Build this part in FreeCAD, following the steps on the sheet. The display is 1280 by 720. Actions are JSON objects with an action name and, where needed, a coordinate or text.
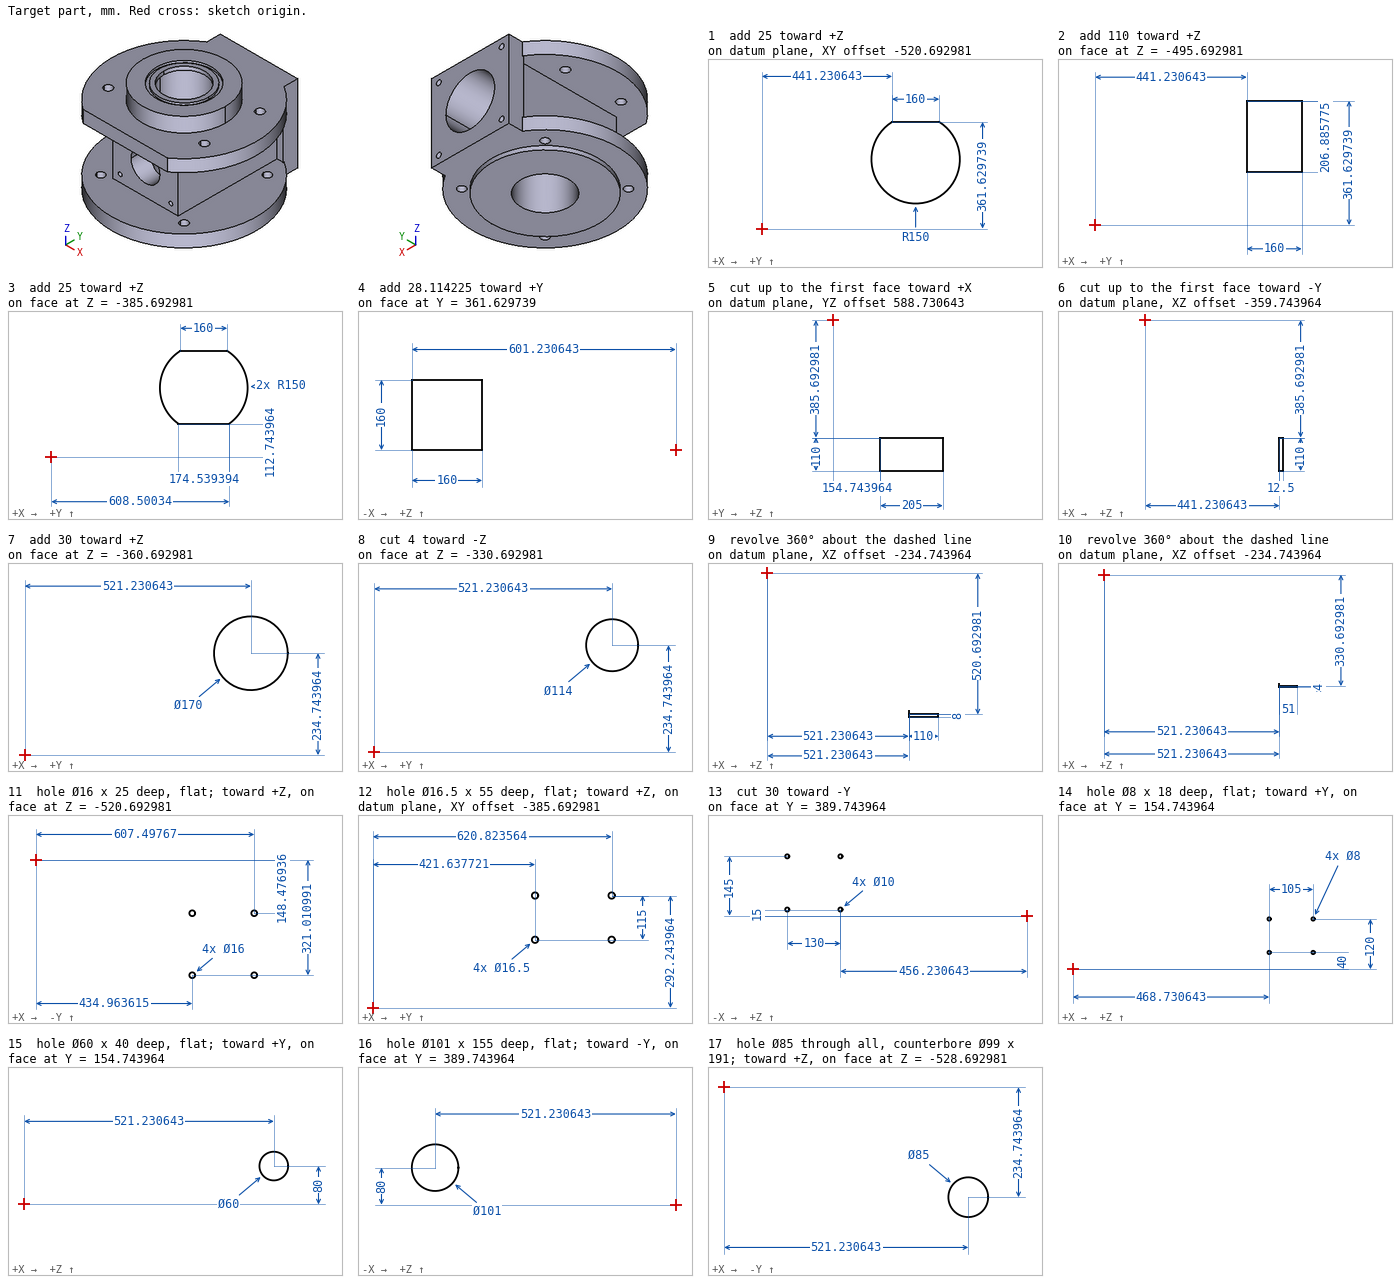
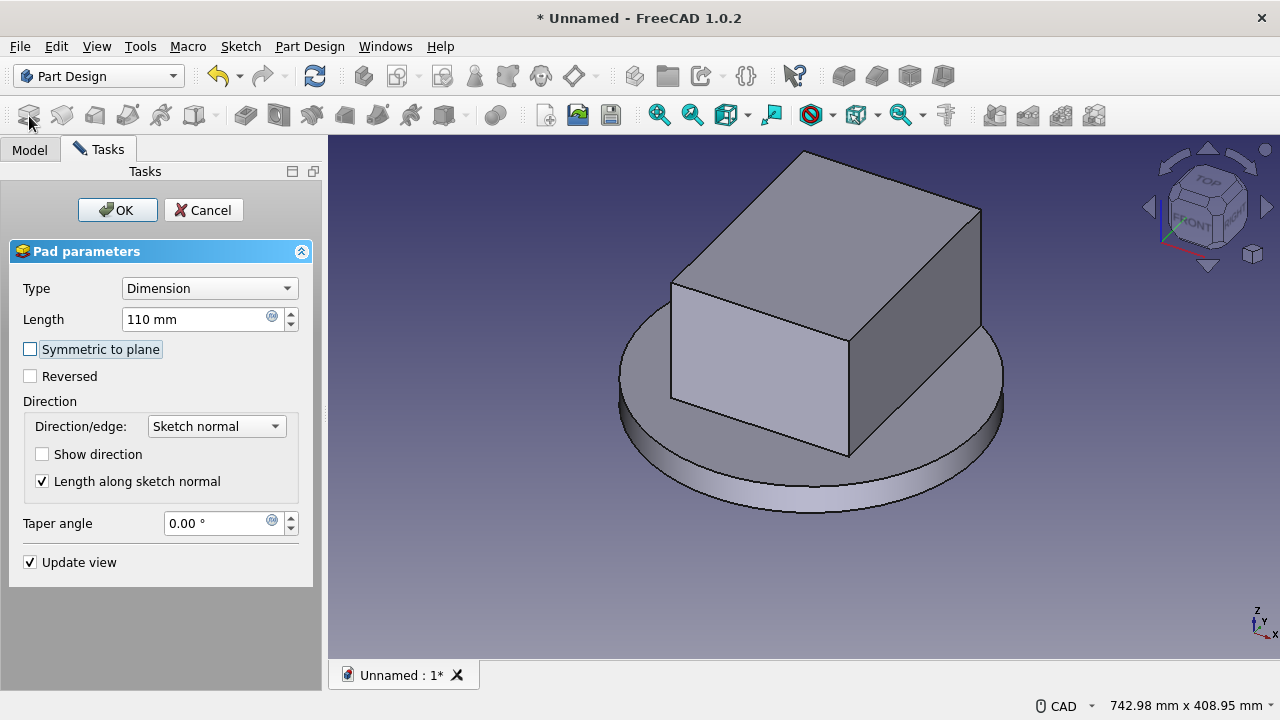
{"action": "left_click", "coordinate": [118, 210]}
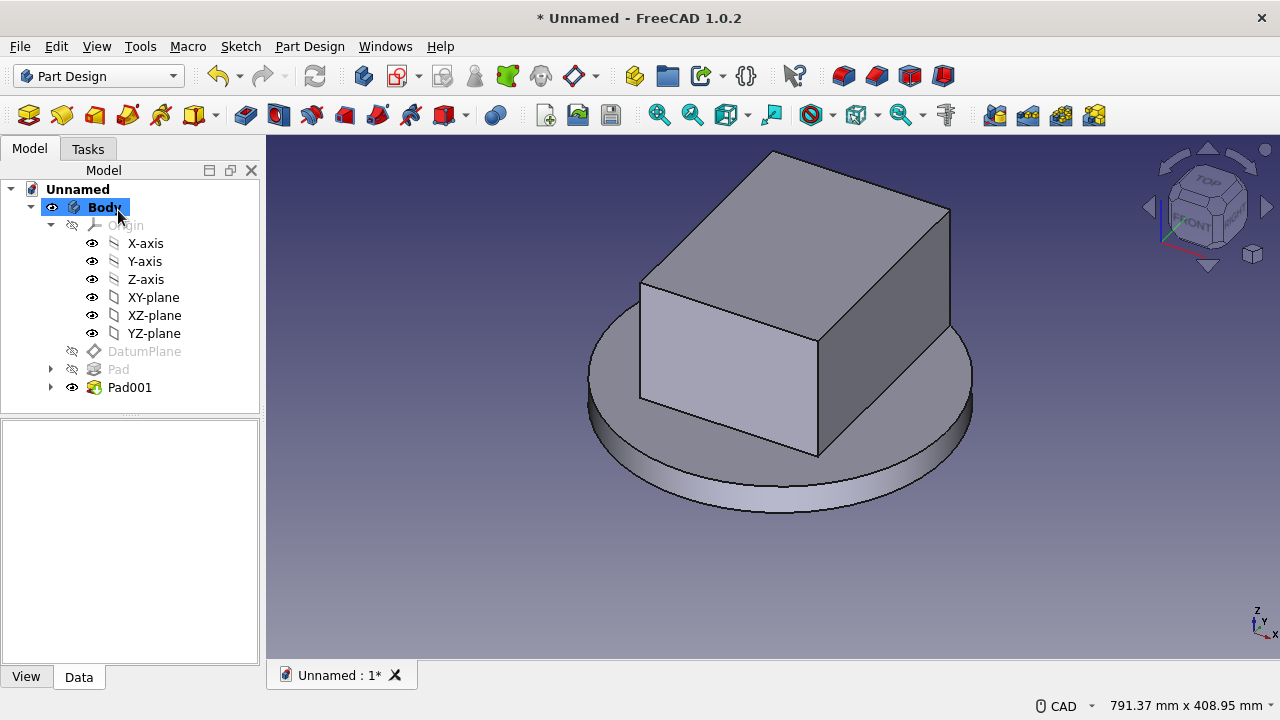
{"action": "left_click", "coordinate": [660, 116]}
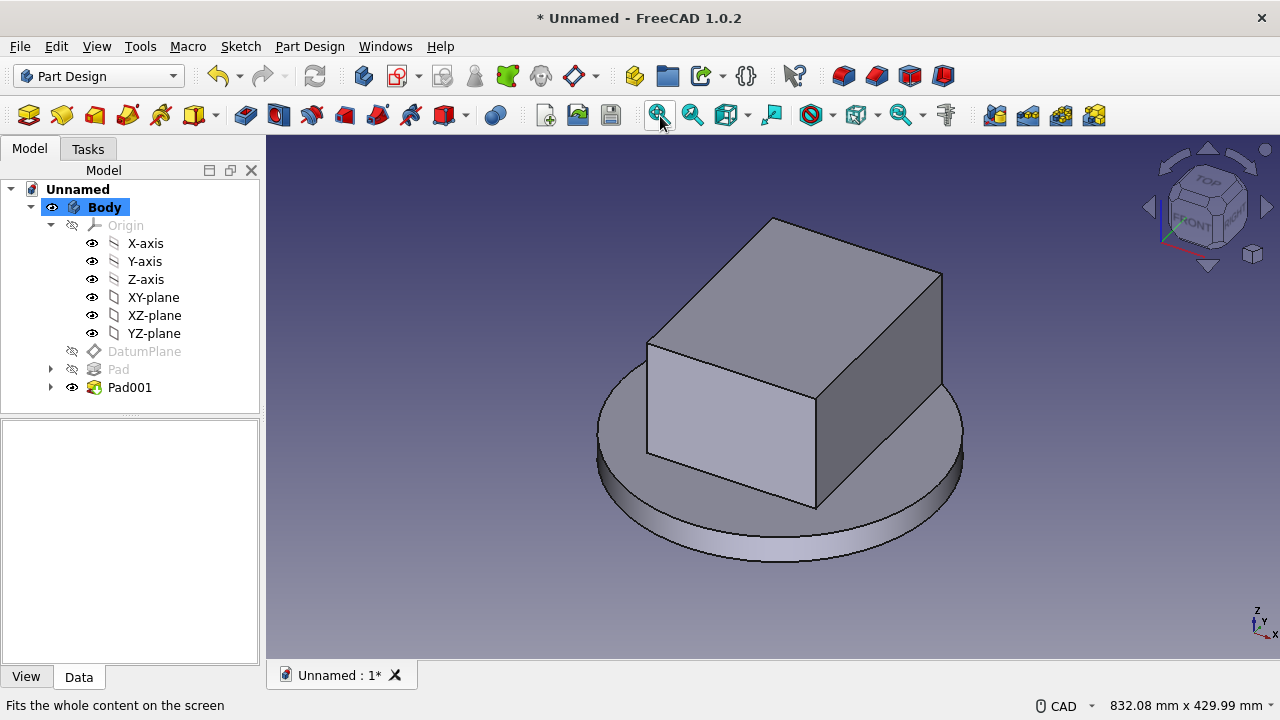
{"action": "left_click", "coordinate": [794, 307]}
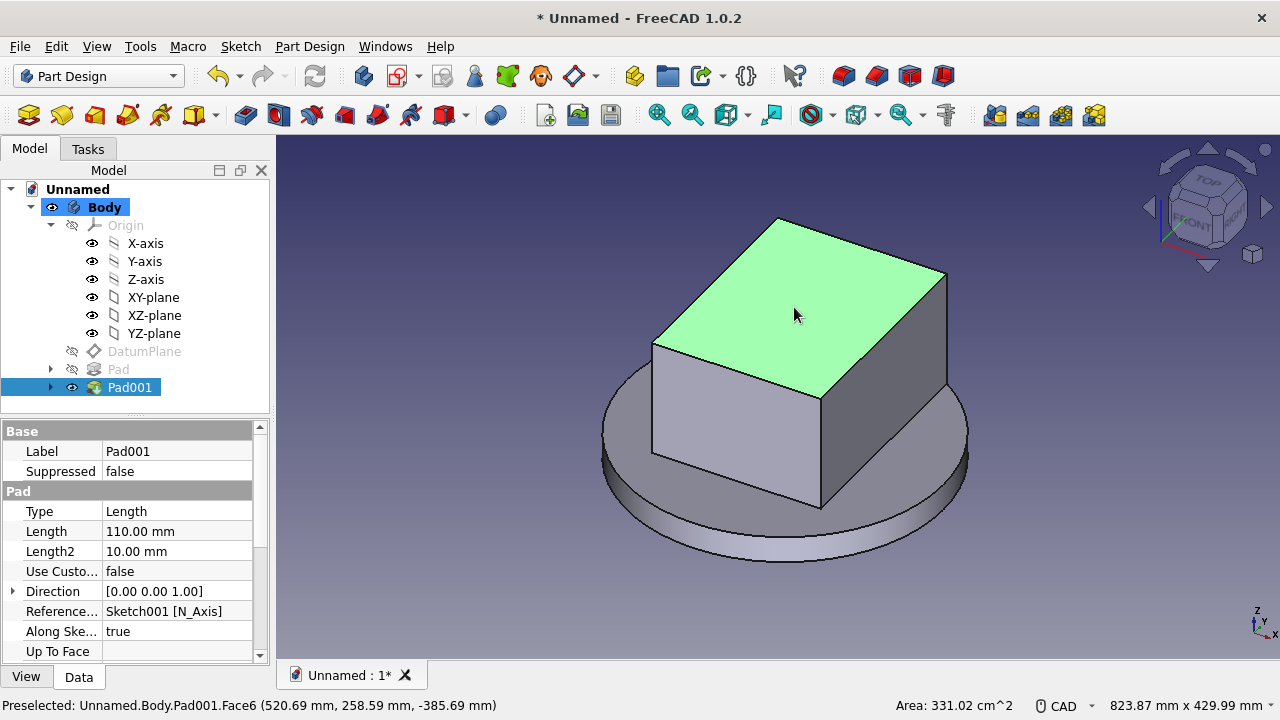
{"action": "left_click", "coordinate": [396, 76]}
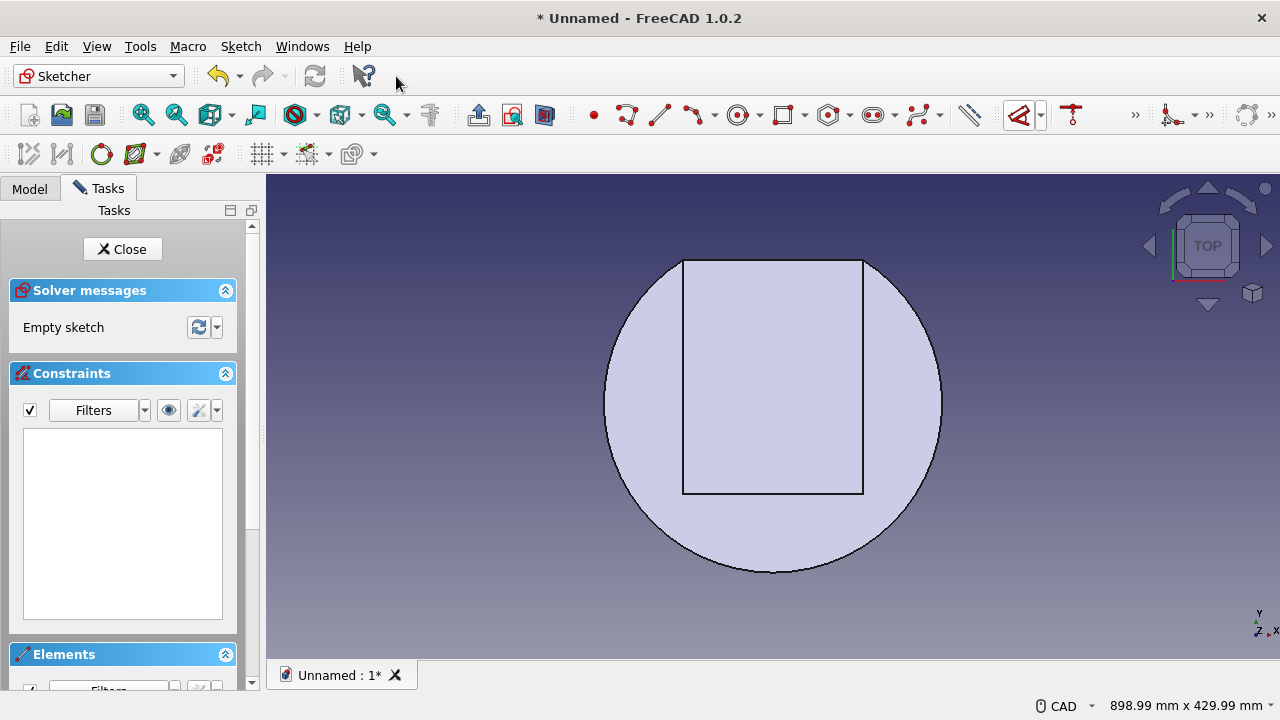
{"action": "scroll", "coordinate": [1115, 202], "scroll_direction": "down", "scroll_amount": 1}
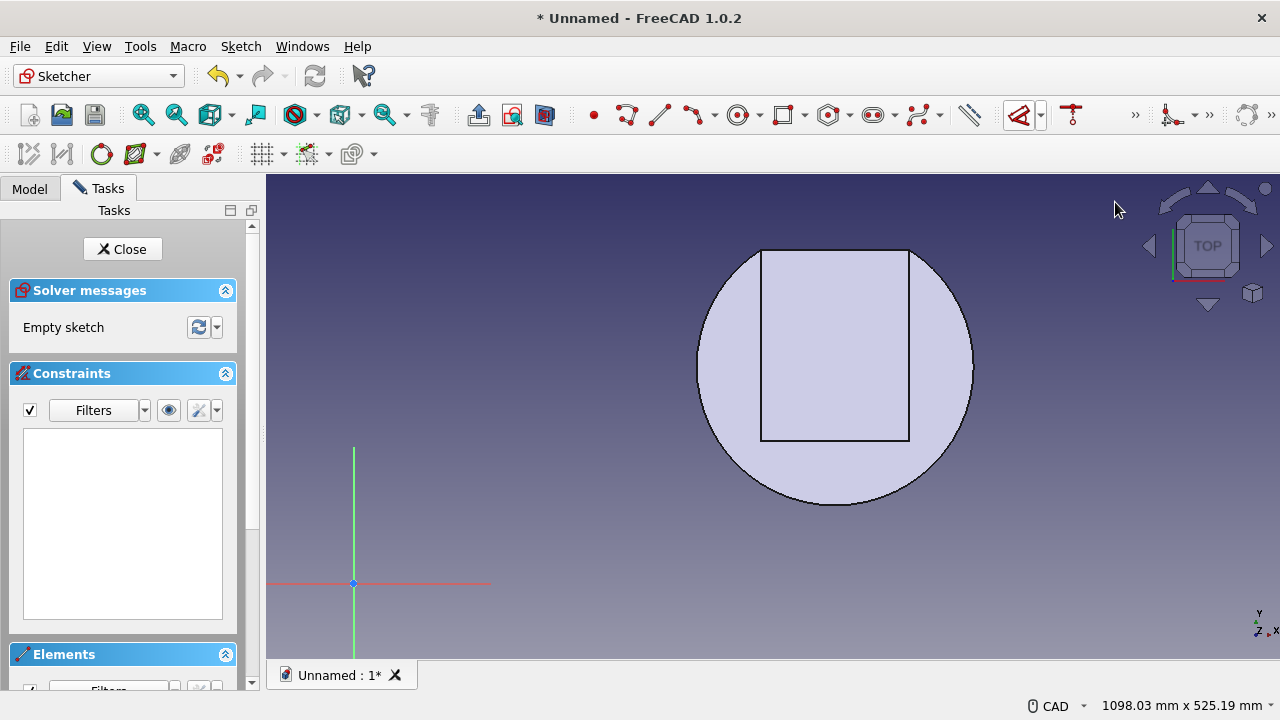
{"action": "left_click", "coordinate": [660, 116]}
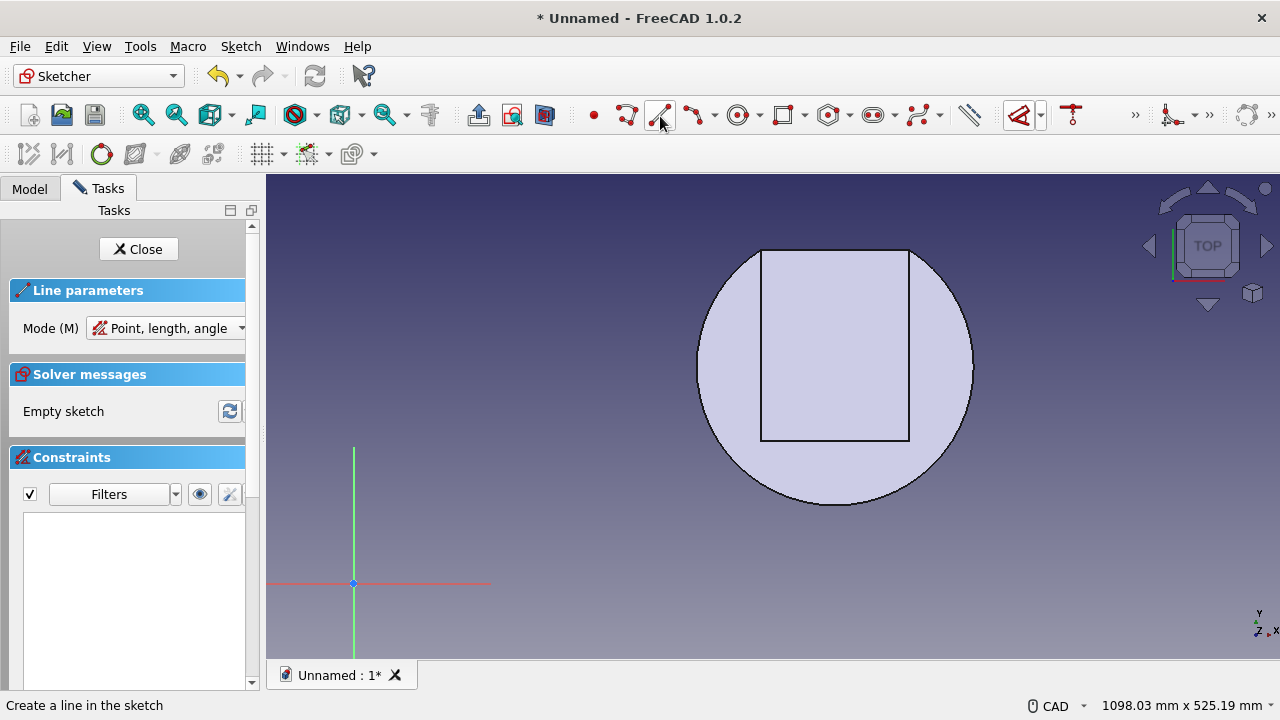
{"action": "left_click", "coordinate": [755, 480]}
{"action": "left_click", "coordinate": [916, 480]}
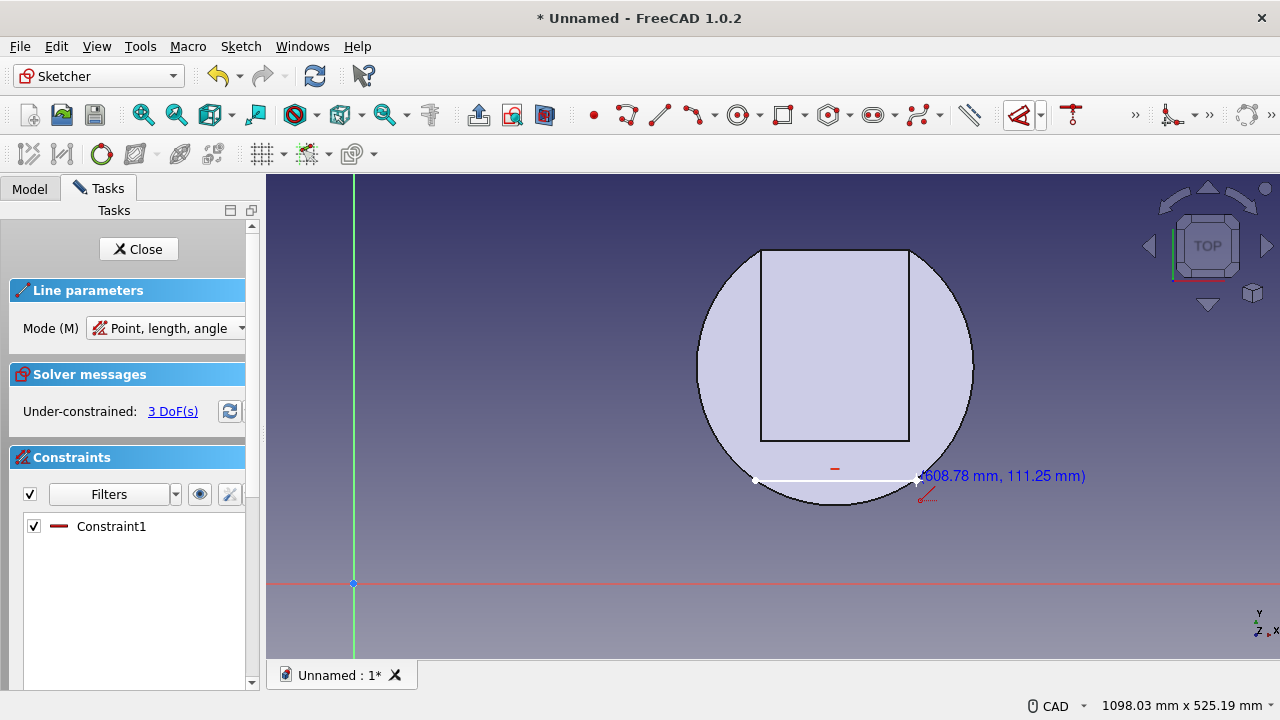
{"action": "left_click", "coordinate": [909, 250]}
{"action": "left_click", "coordinate": [761, 250]}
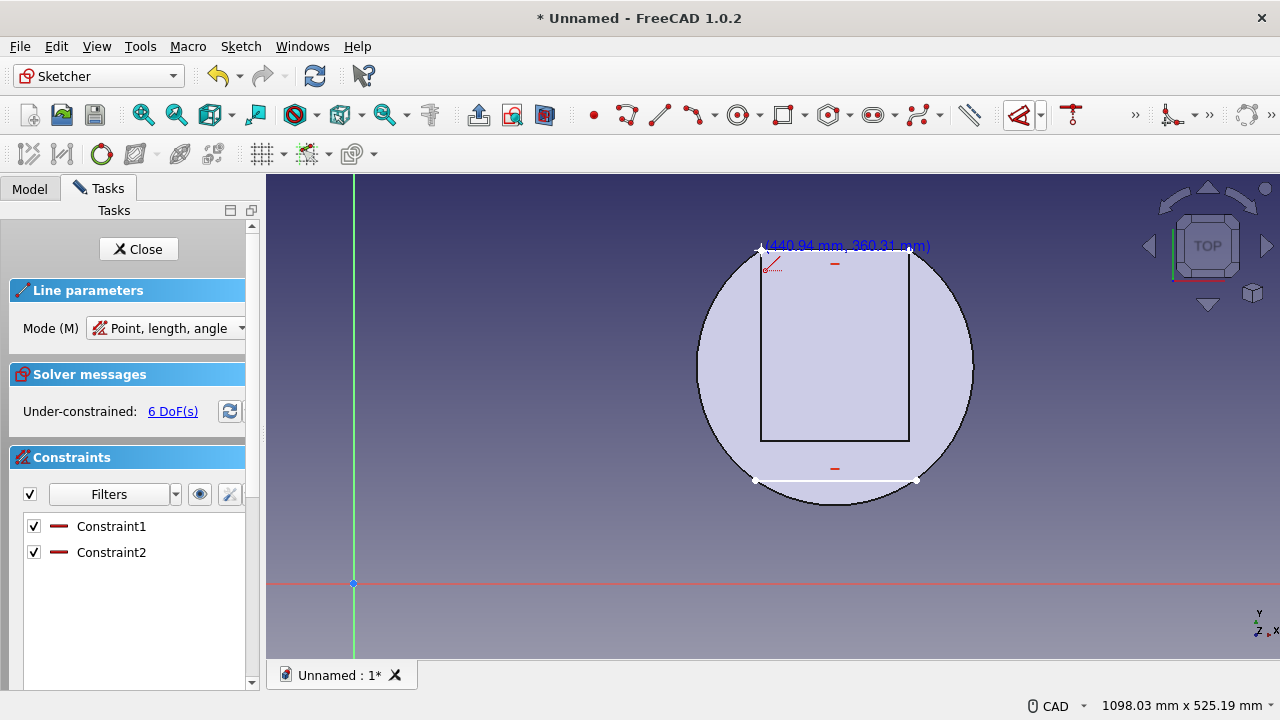
{"action": "left_click", "coordinate": [692, 116]}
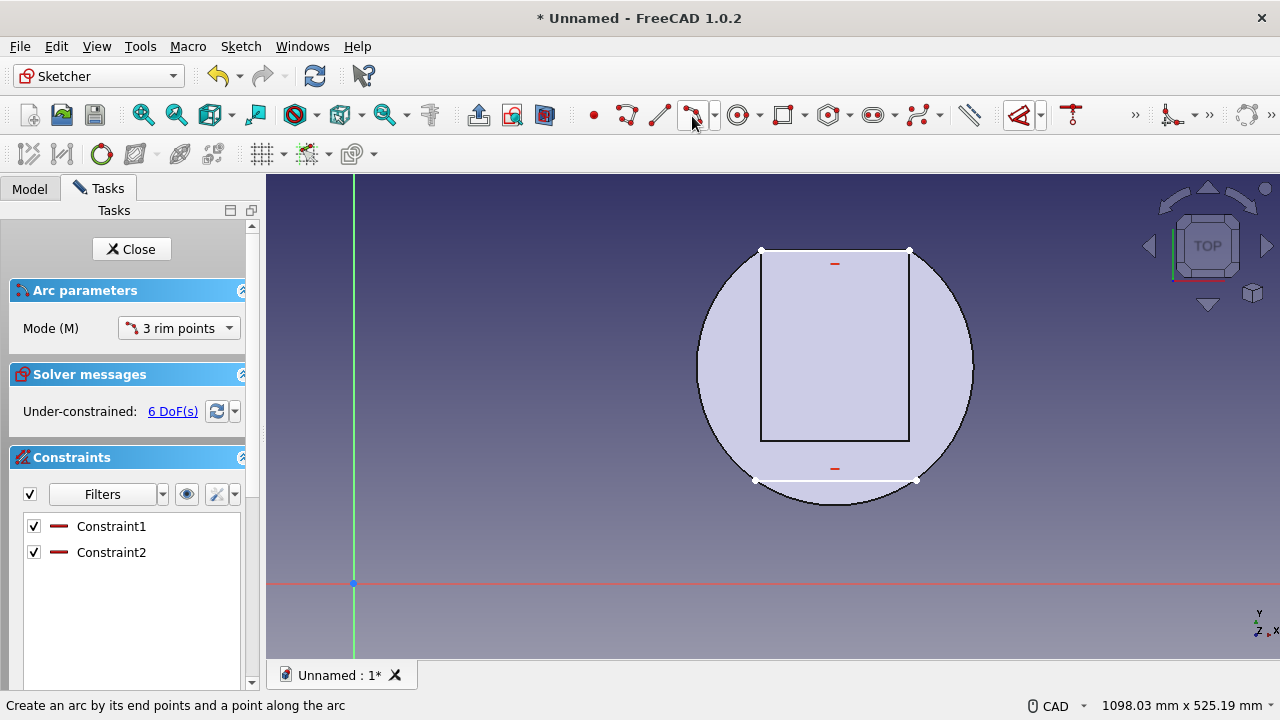
{"action": "left_click", "coordinate": [916, 481]}
{"action": "left_click", "coordinate": [909, 251]}
{"action": "left_click", "coordinate": [974, 363]}